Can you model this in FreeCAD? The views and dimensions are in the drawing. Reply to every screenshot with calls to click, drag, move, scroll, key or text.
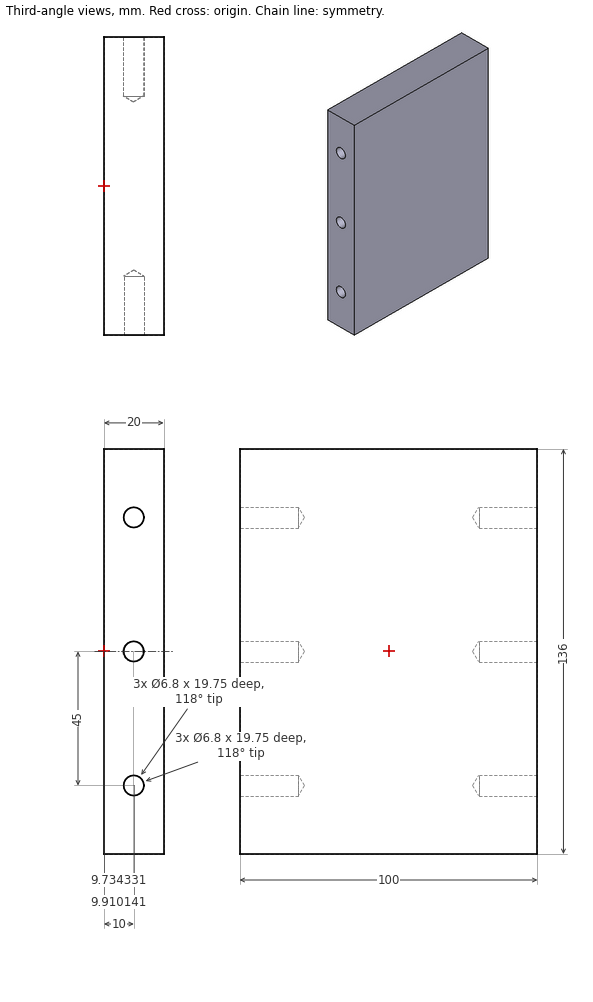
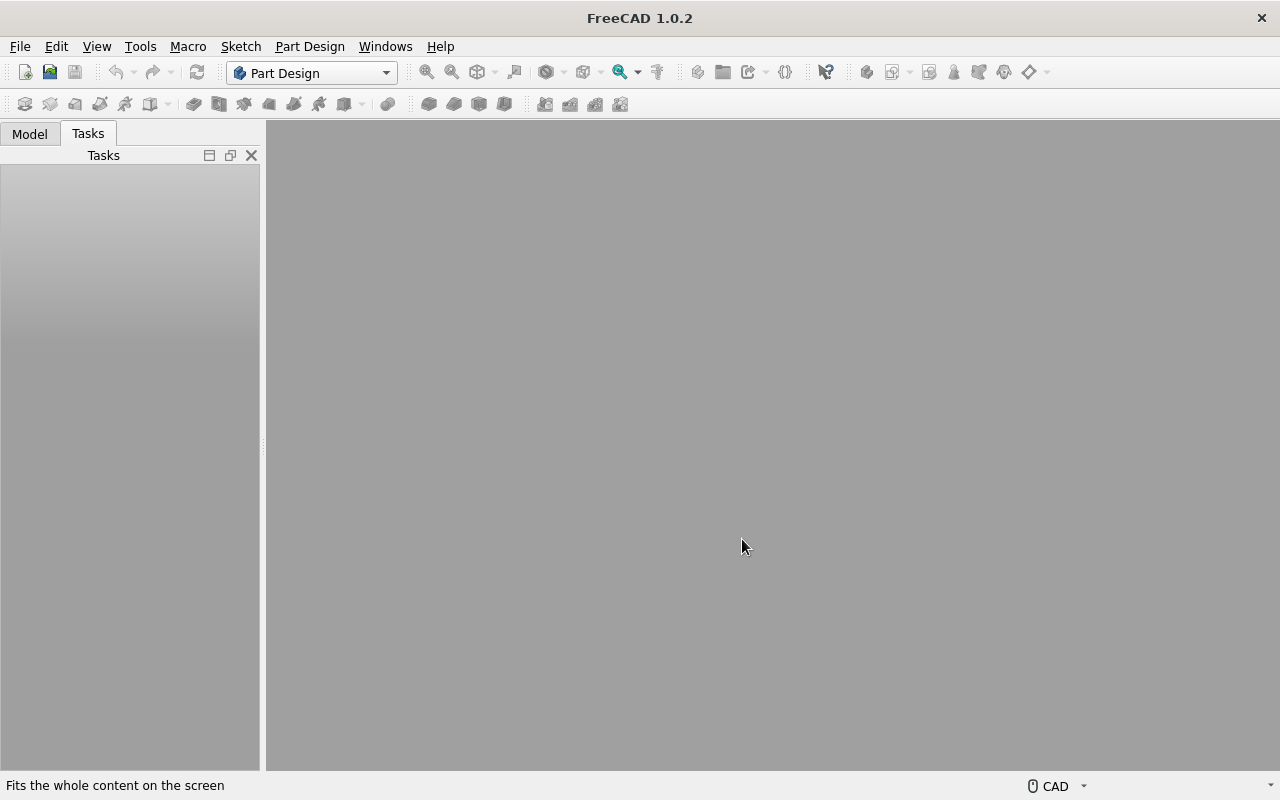
click(25, 72)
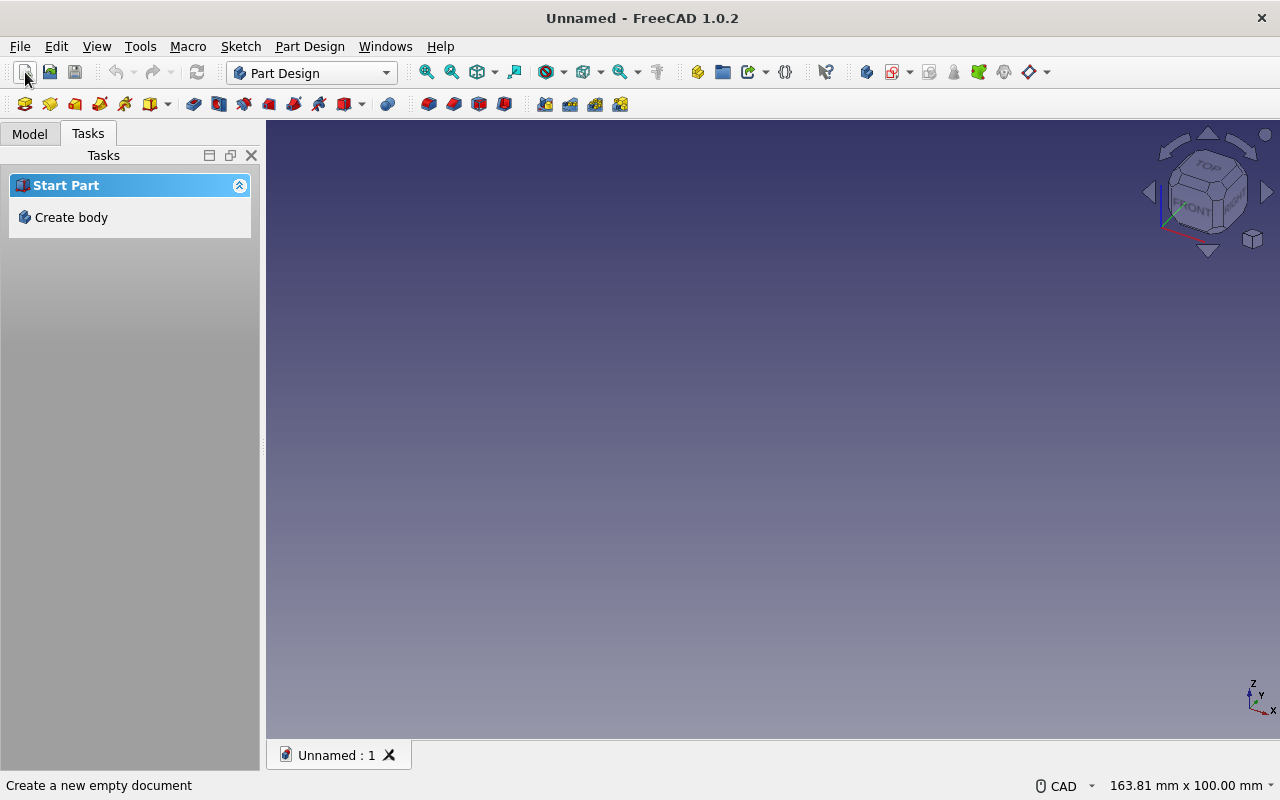
click(892, 72)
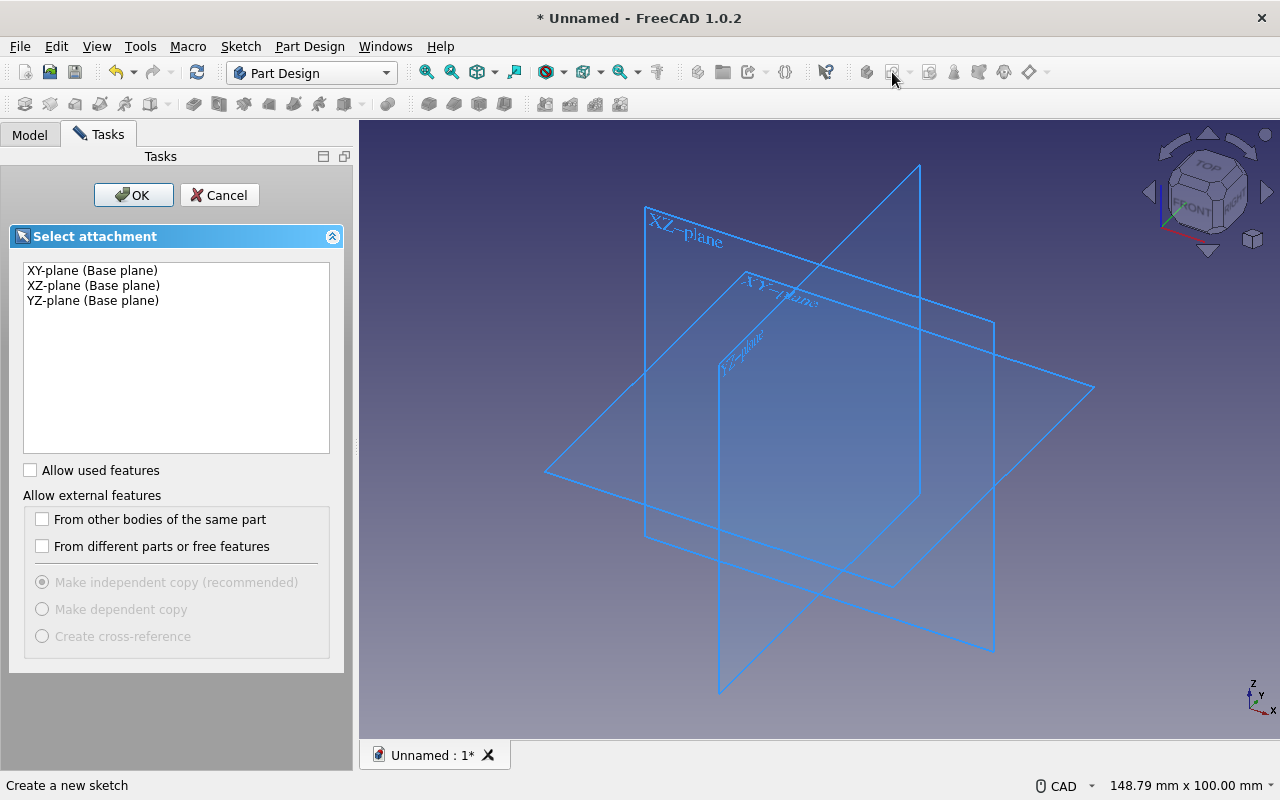
click(84, 300)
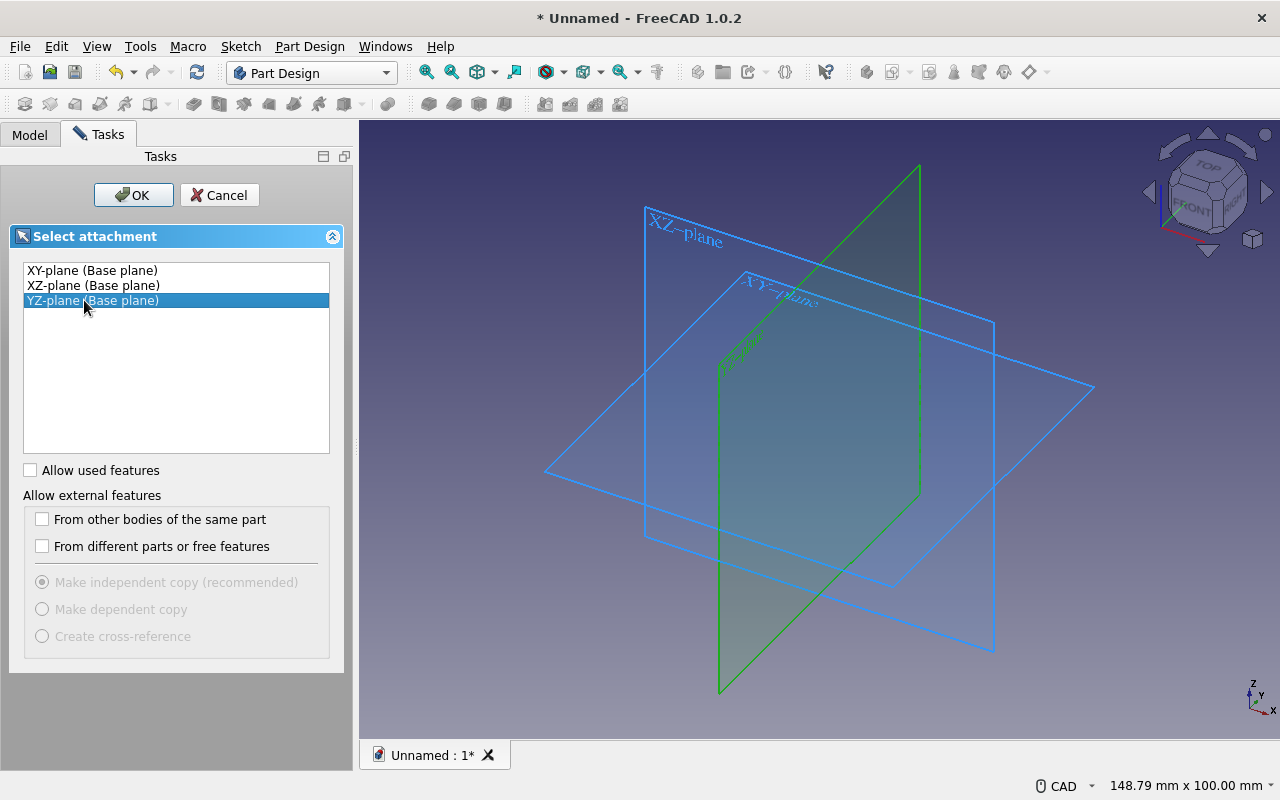
click(134, 195)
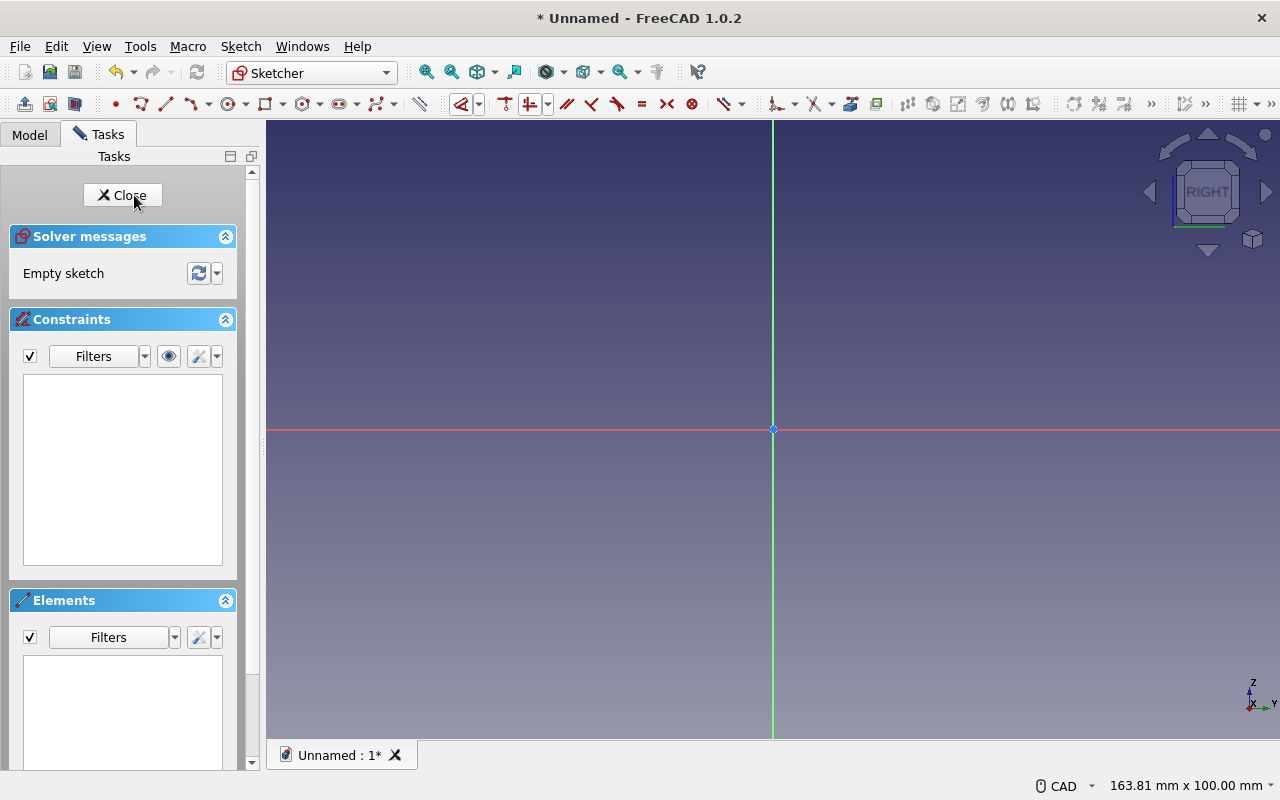
scroll(649, 430, down, 4)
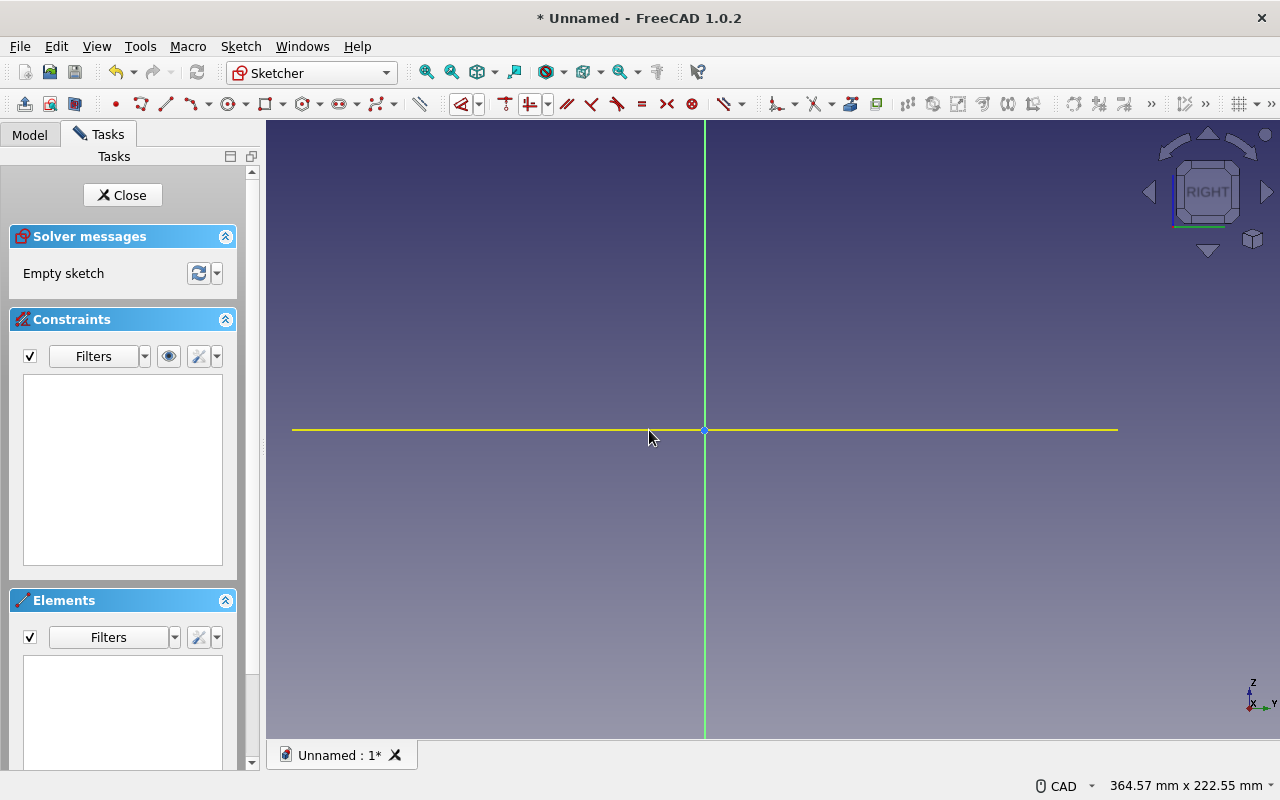
key(g)
key(v)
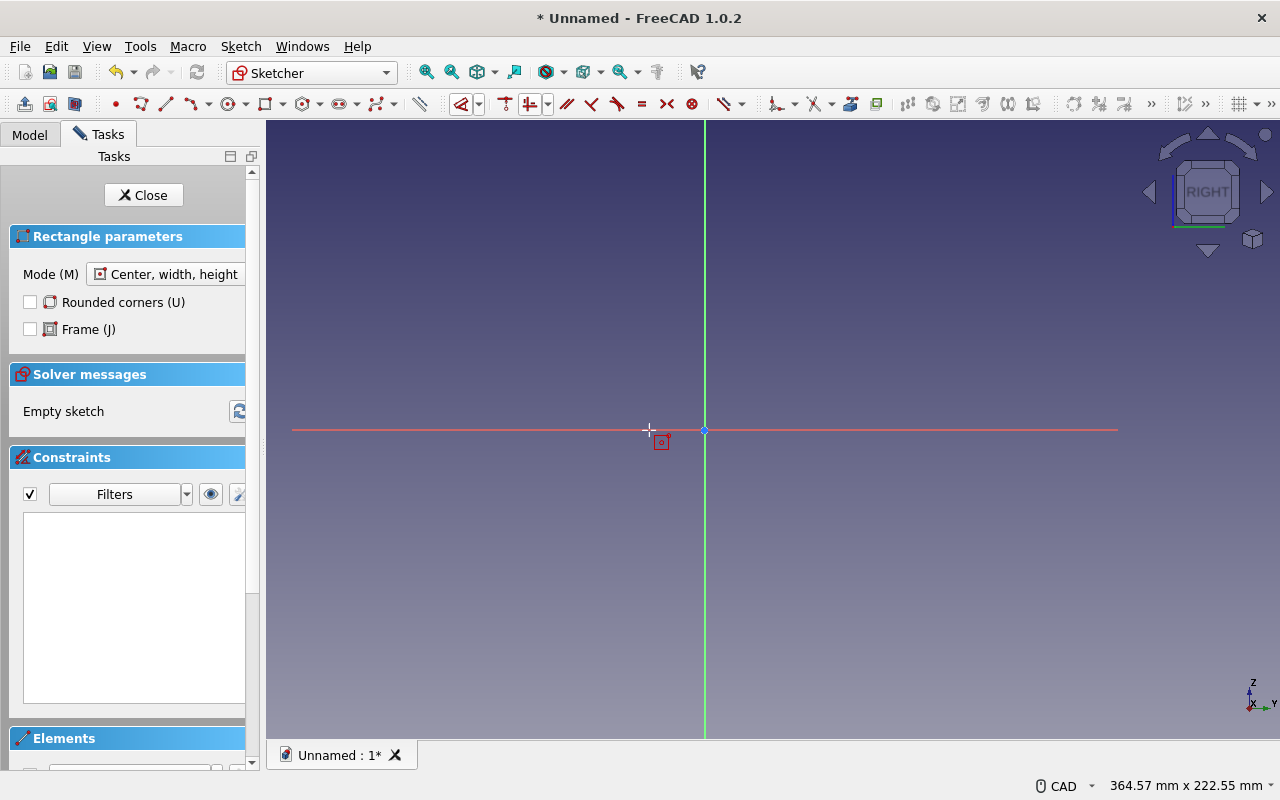
click(705, 430)
click(844, 241)
key(Escape)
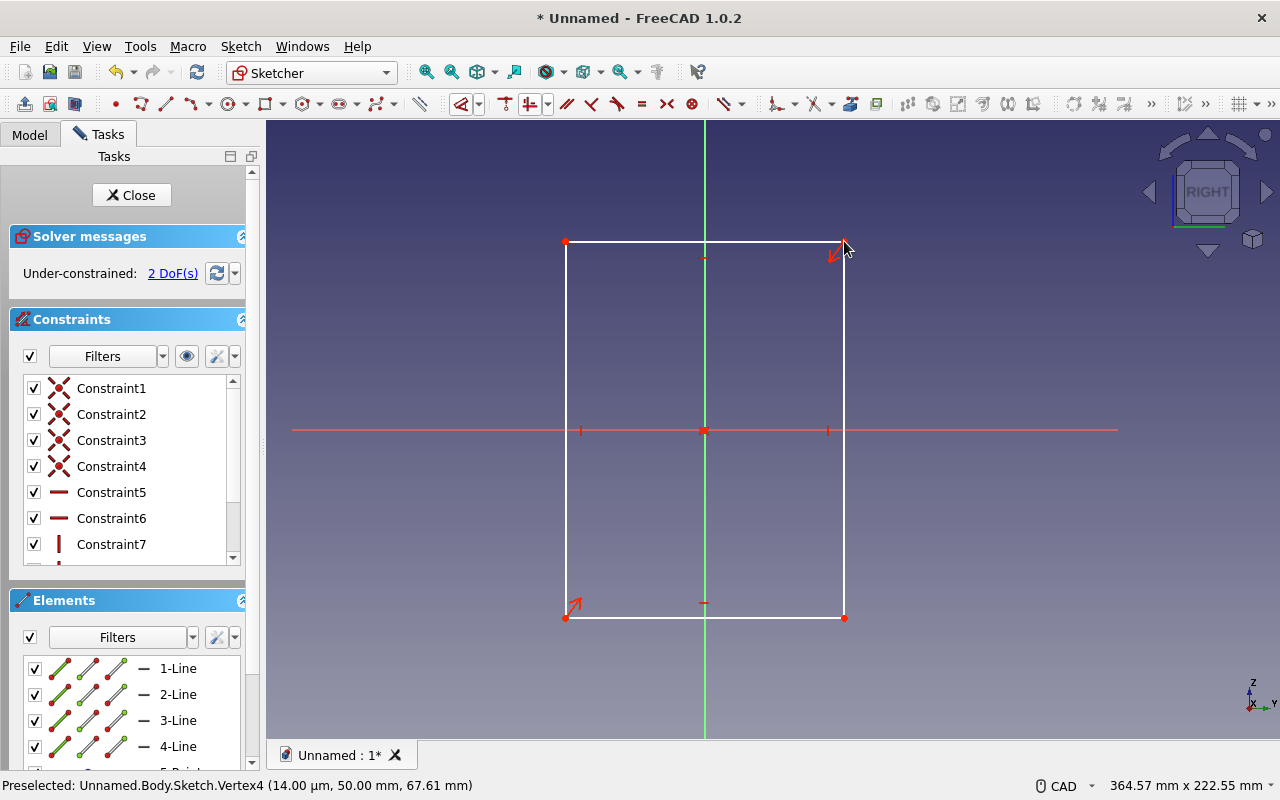
click(649, 618)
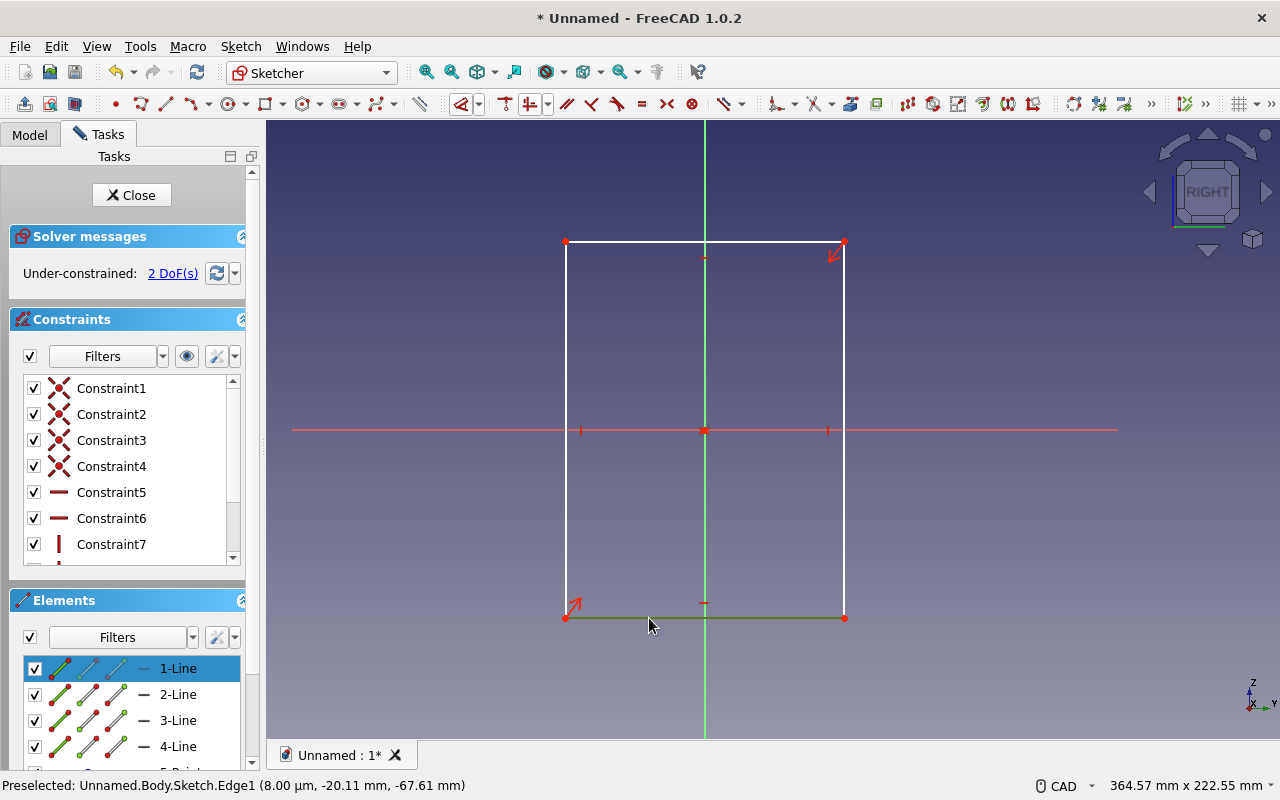
click(478, 104)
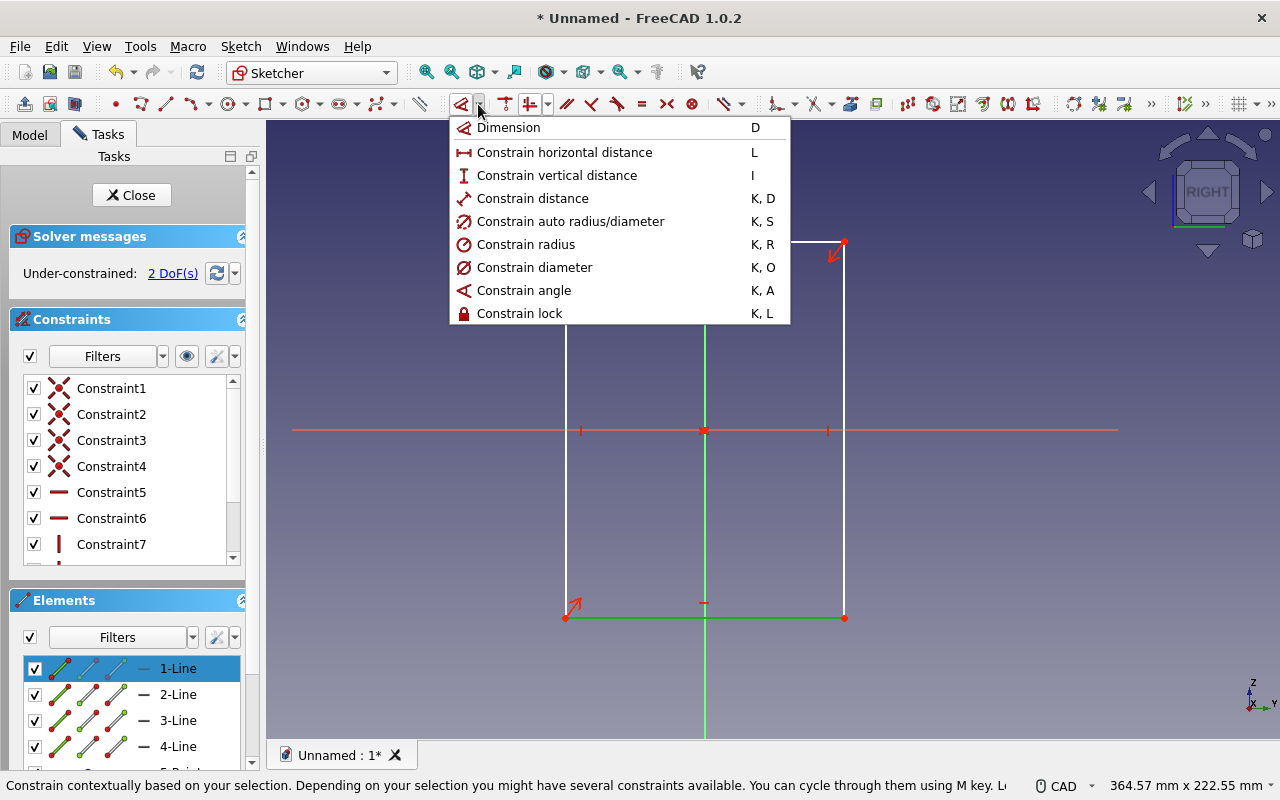
click(620, 152)